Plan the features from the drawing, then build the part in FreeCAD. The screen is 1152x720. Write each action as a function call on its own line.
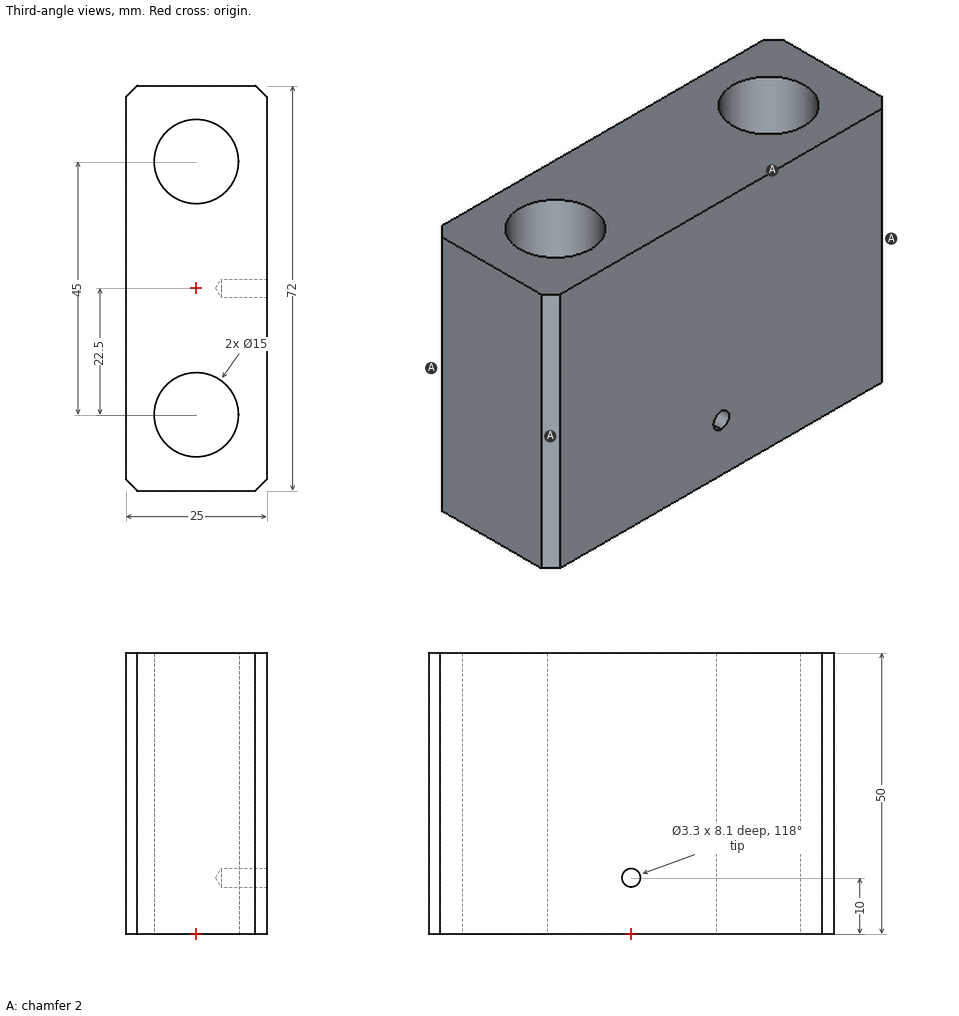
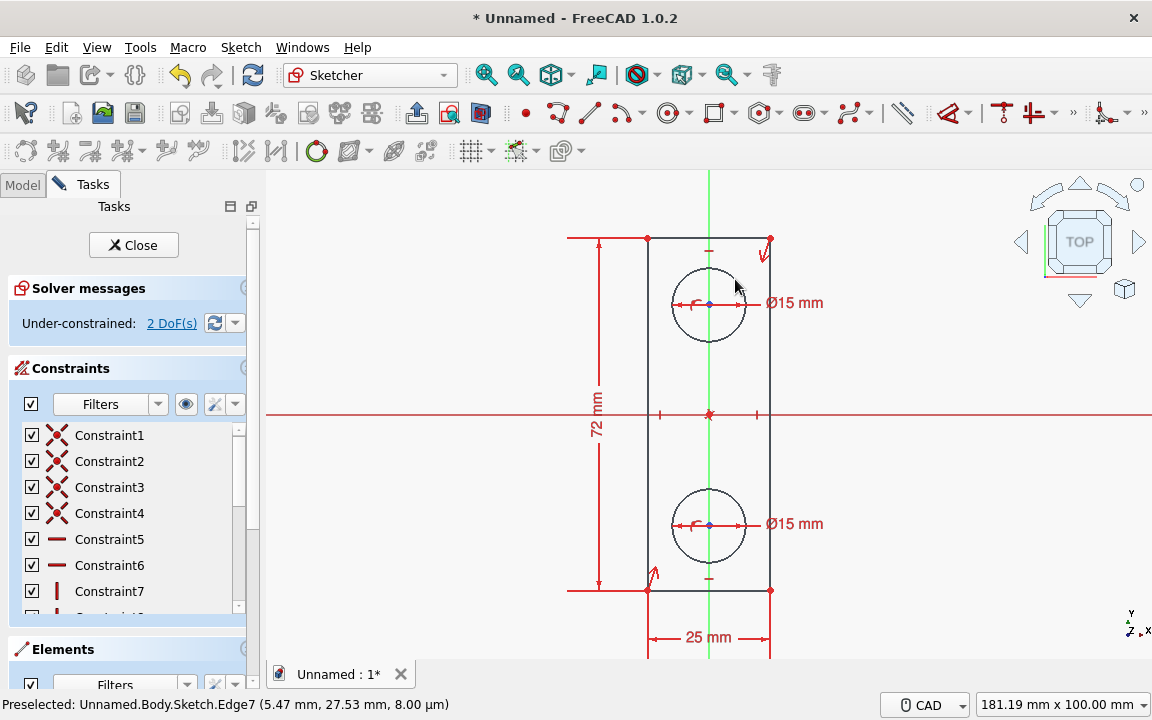
click(709, 526)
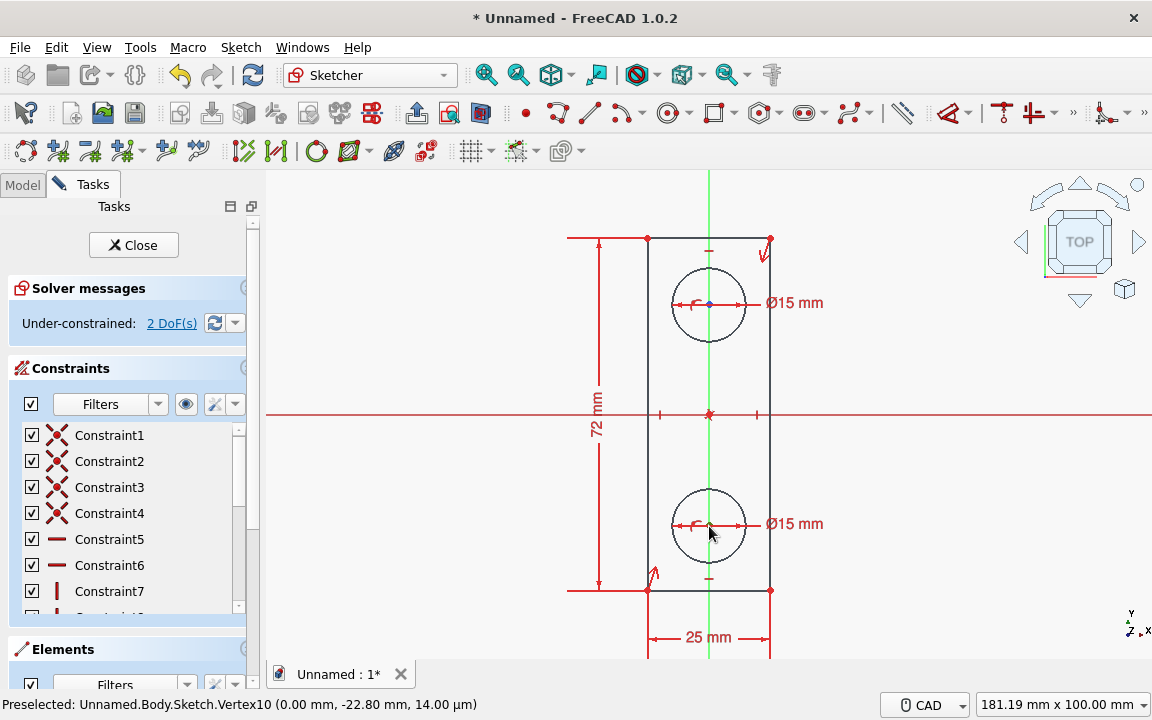
click(709, 305)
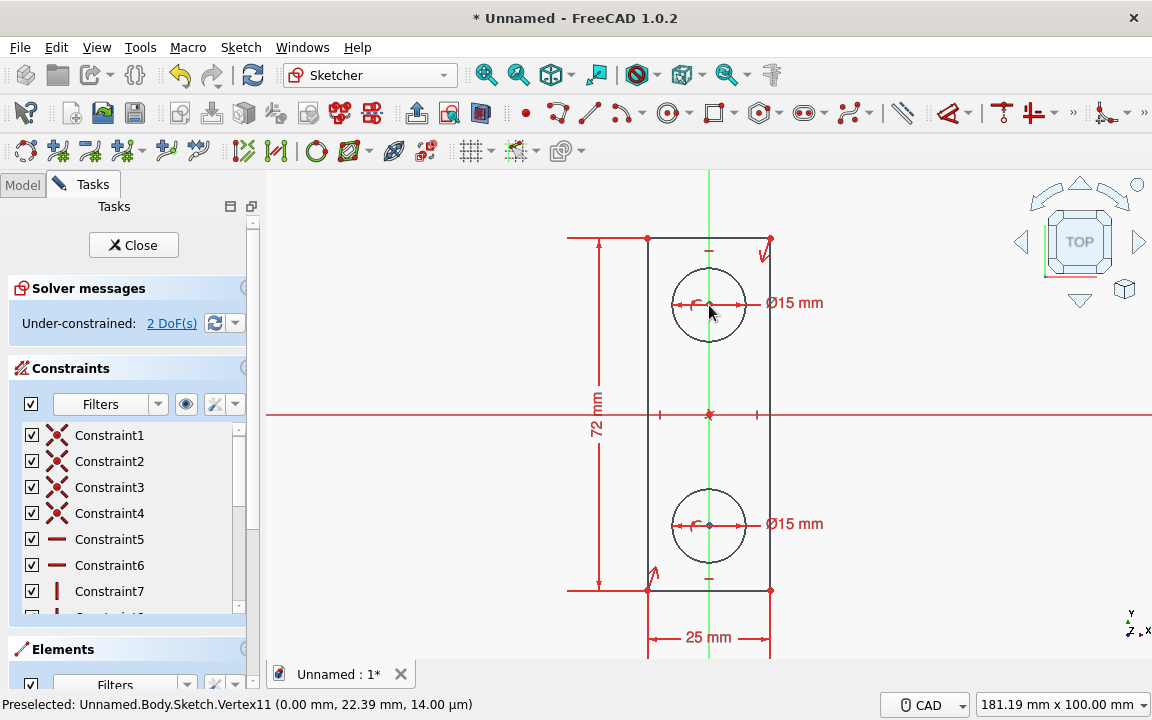
key(i)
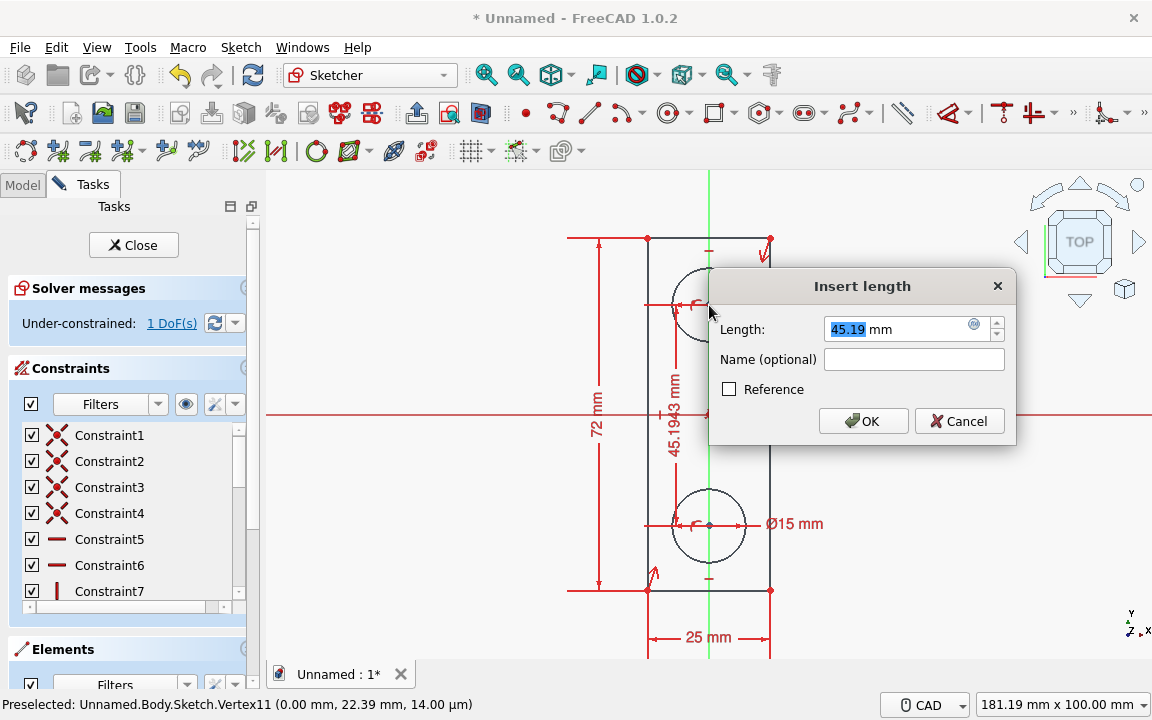
text(45)
key(Return)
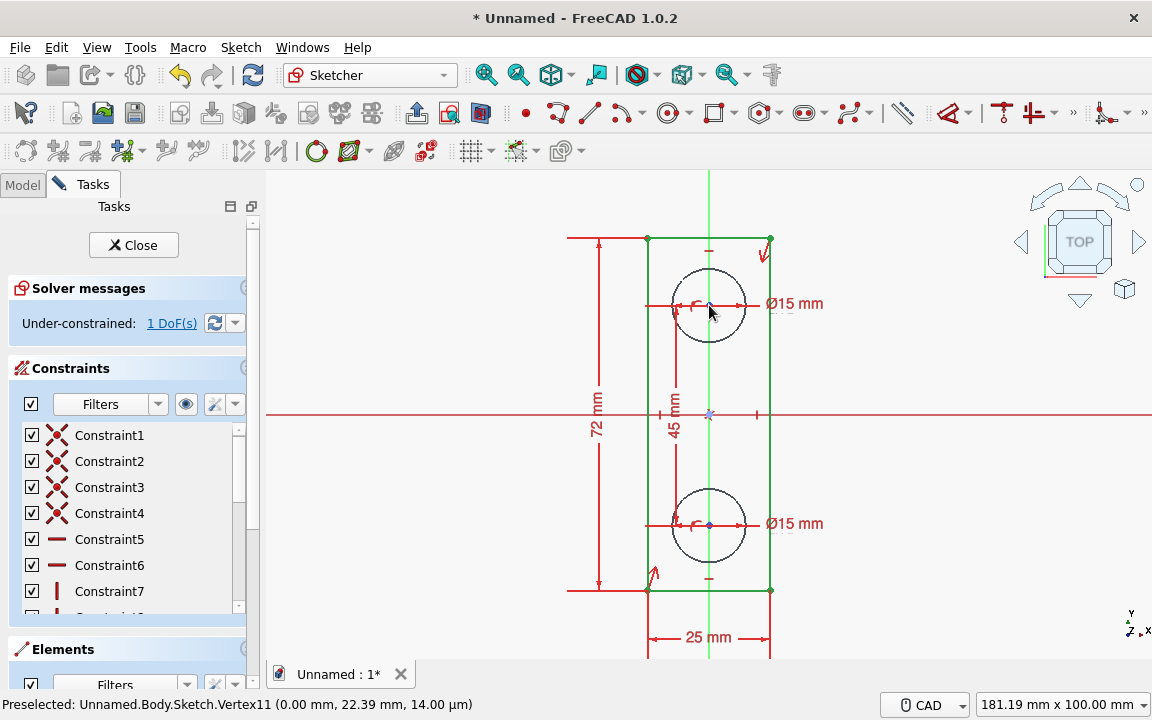
click(709, 526)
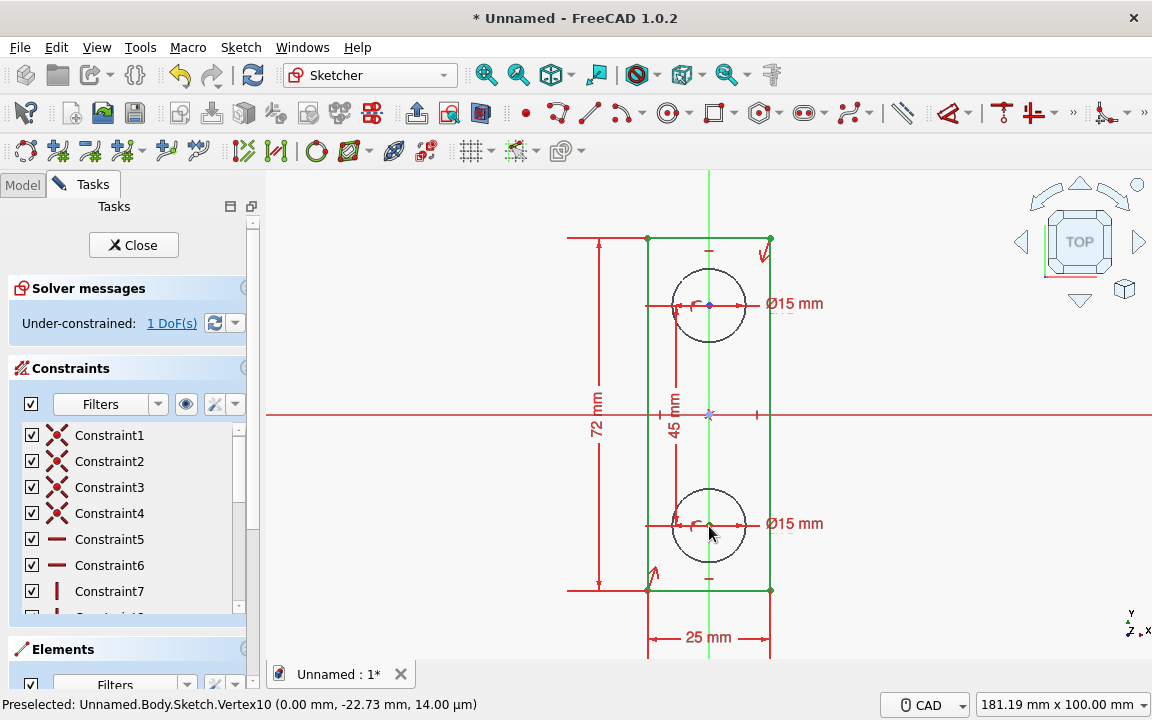
click(970, 114)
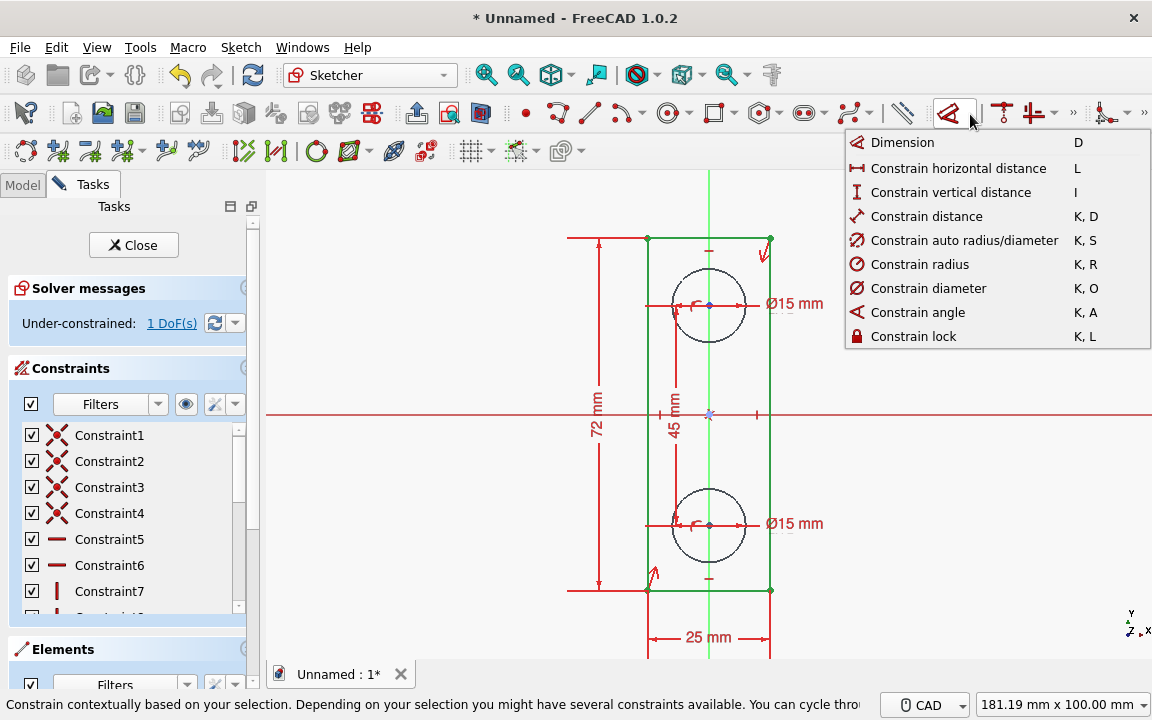
click(998, 192)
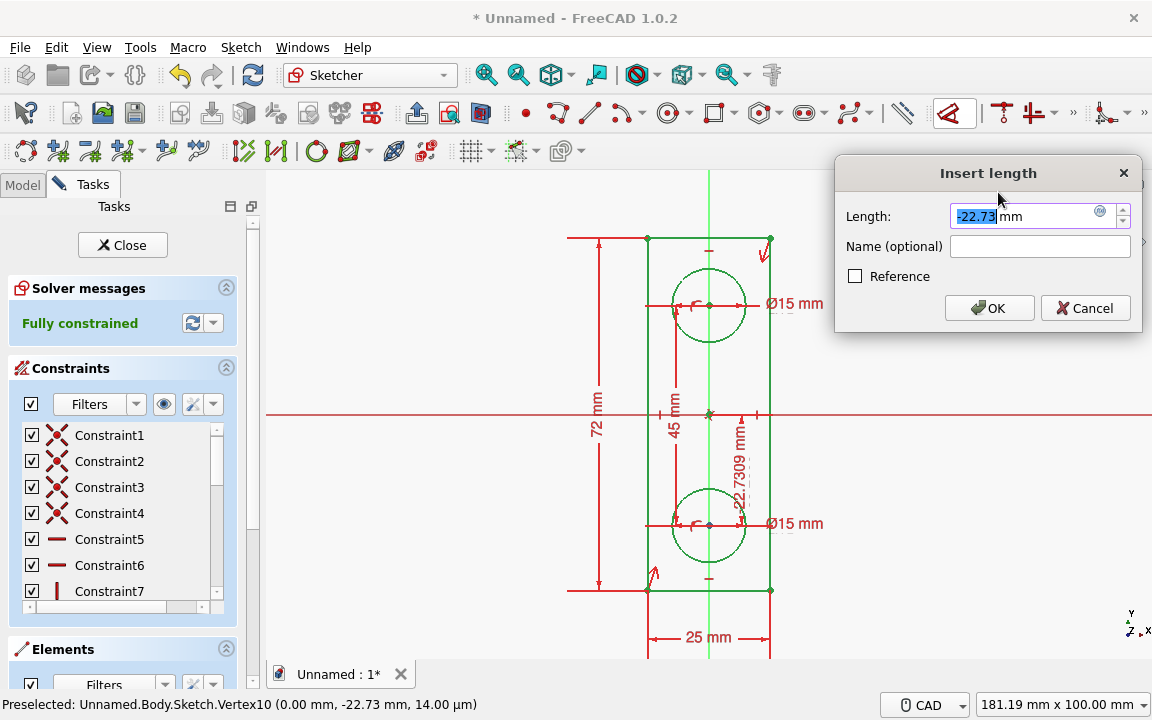
text(-22.5)
key(Return)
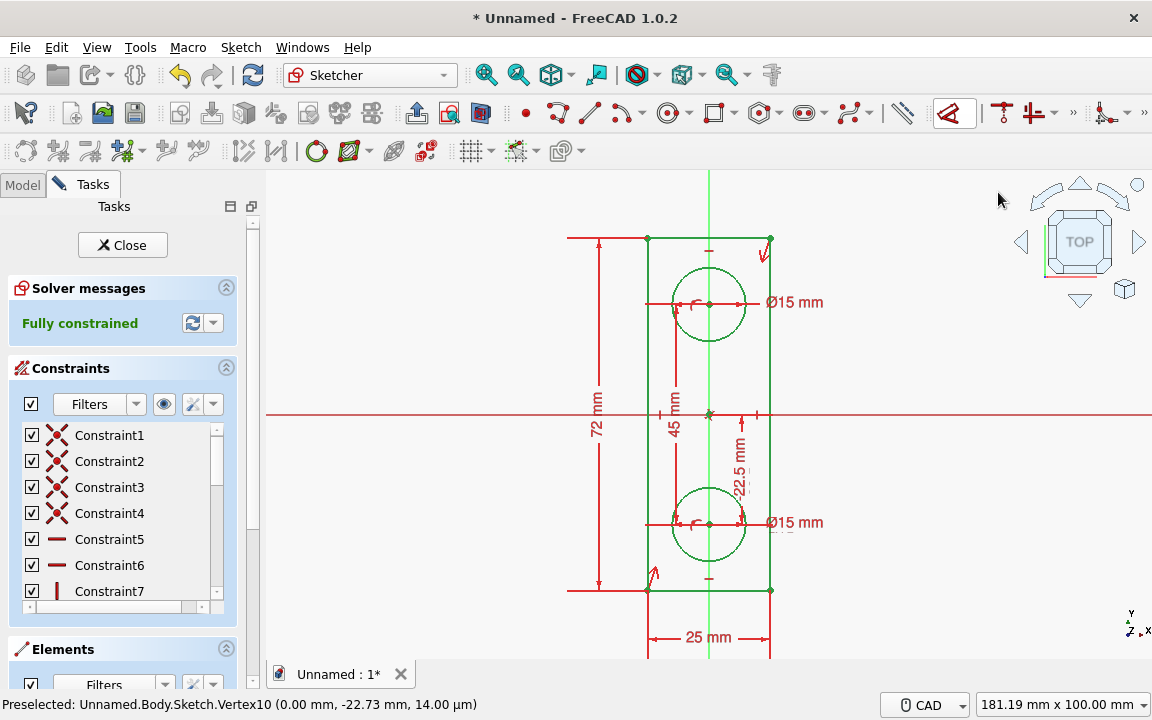
click(123, 245)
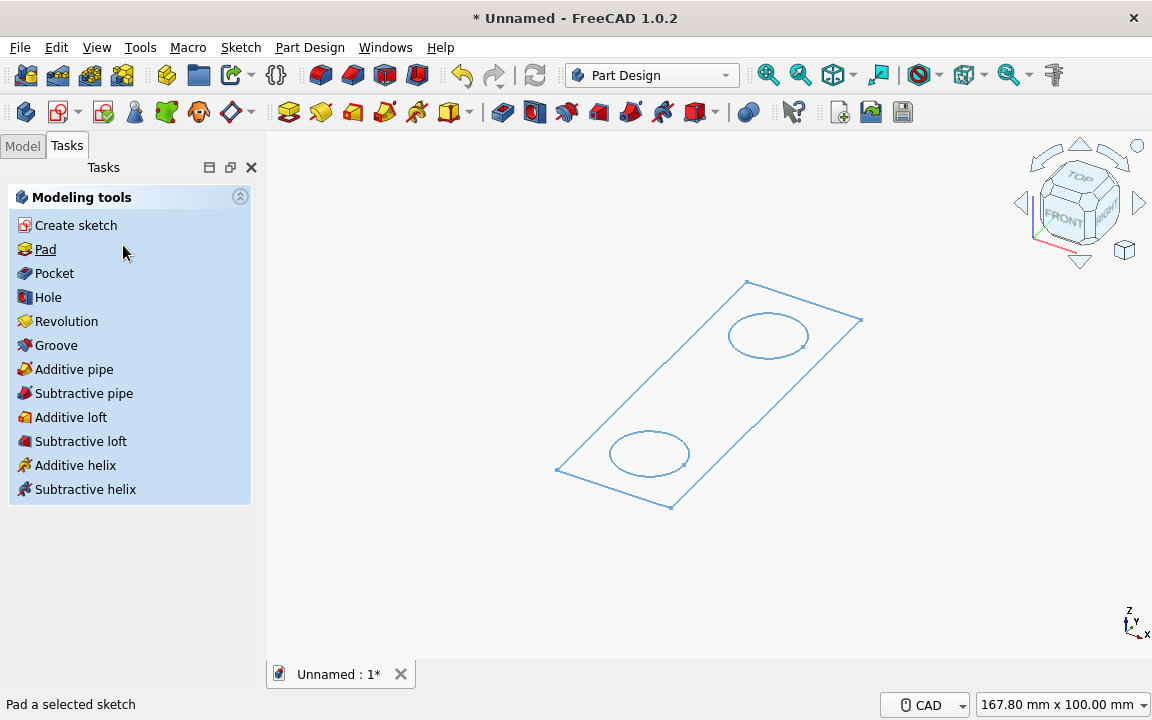
click(290, 112)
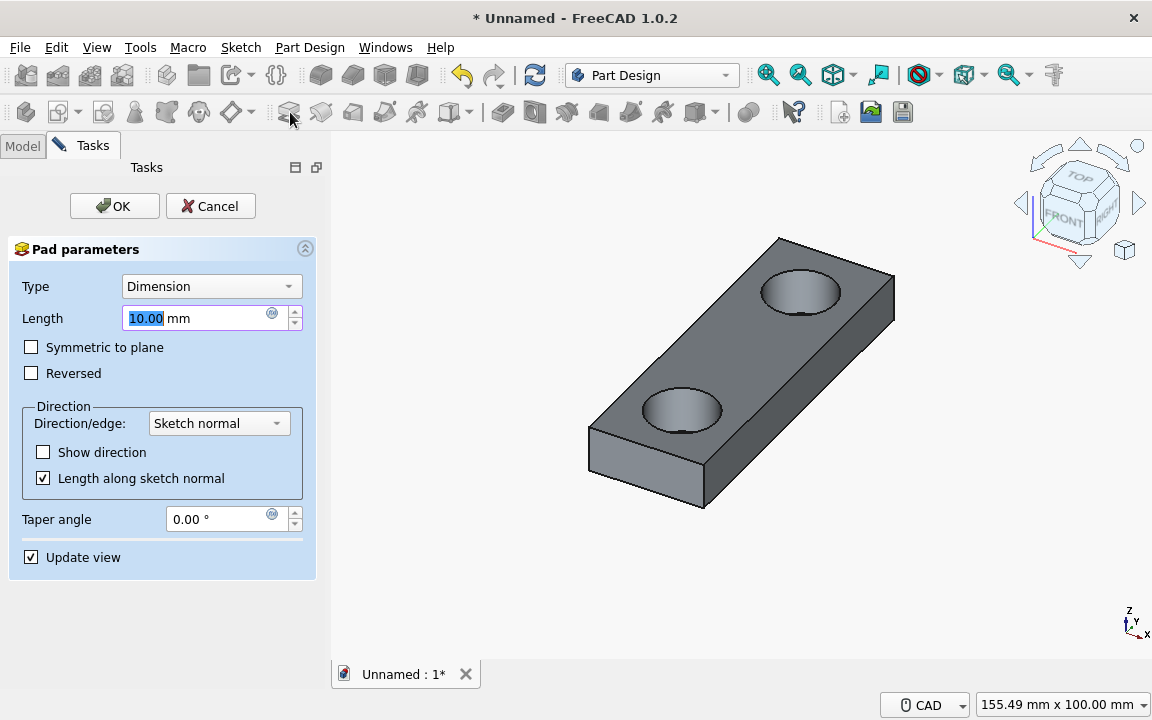
text(50)
key(Tab)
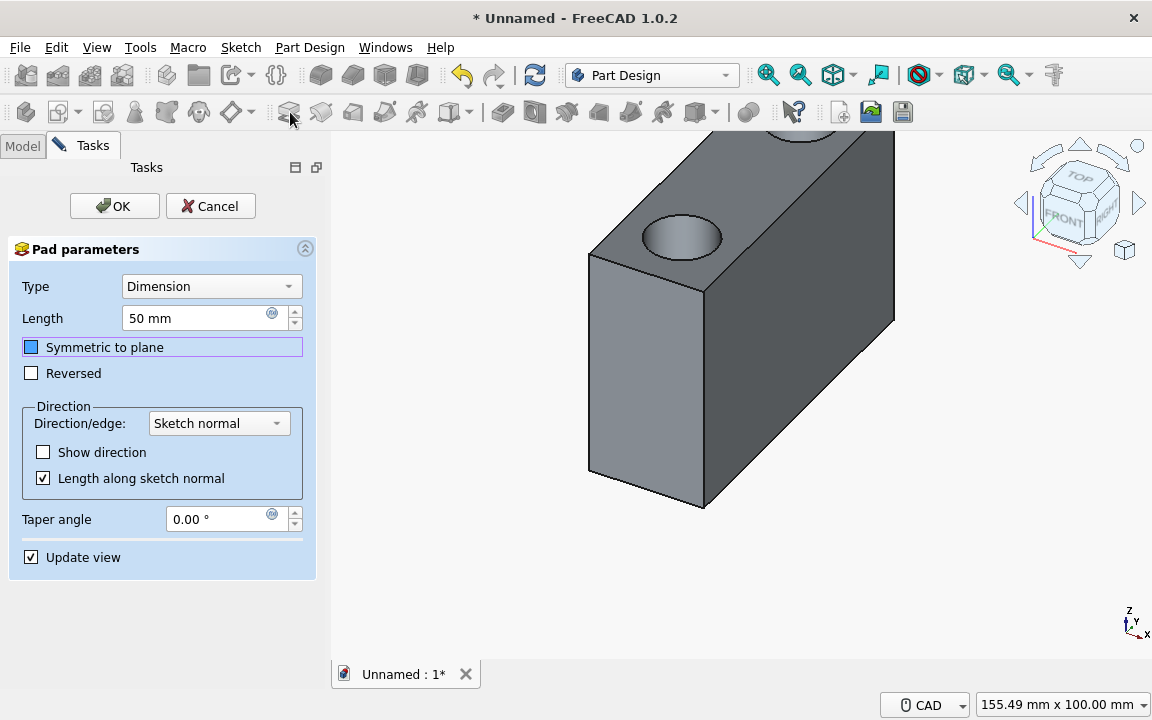
click(115, 206)